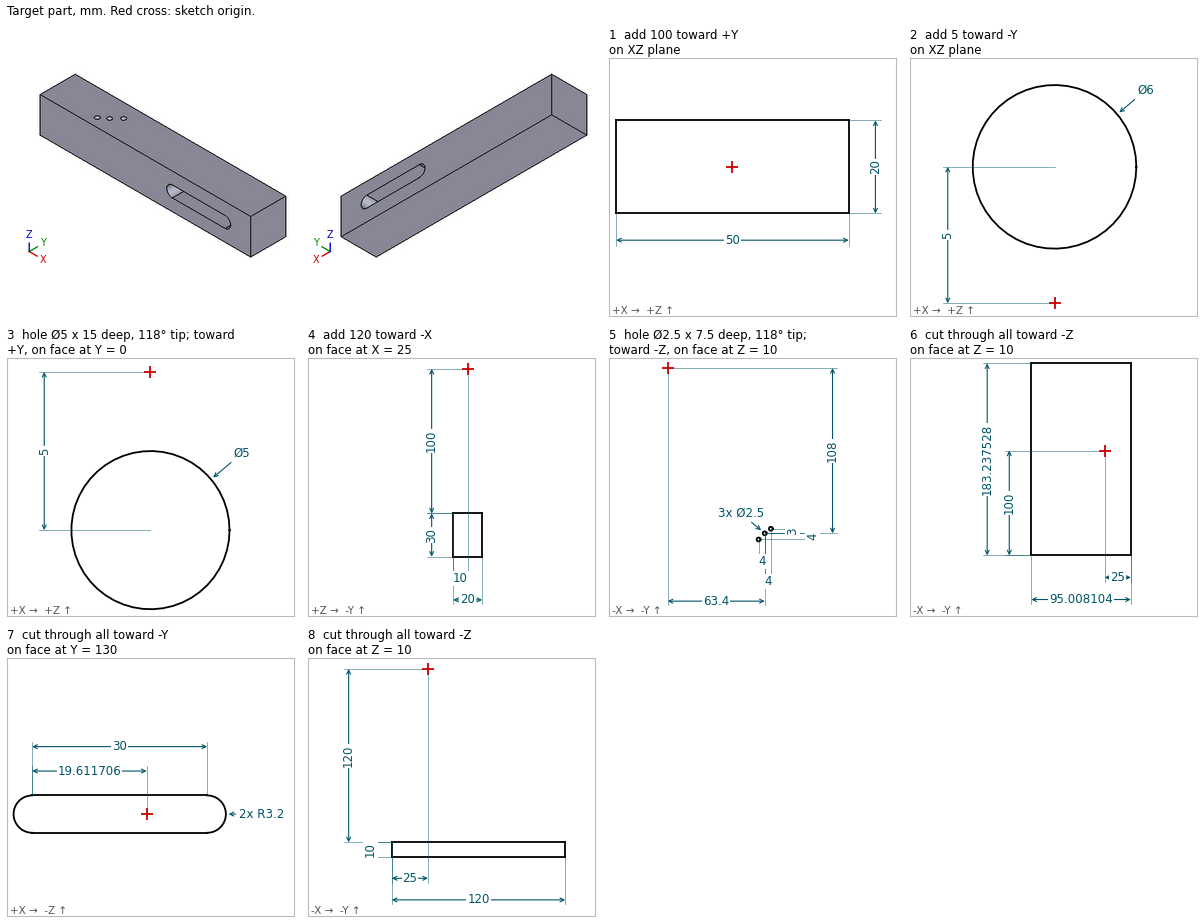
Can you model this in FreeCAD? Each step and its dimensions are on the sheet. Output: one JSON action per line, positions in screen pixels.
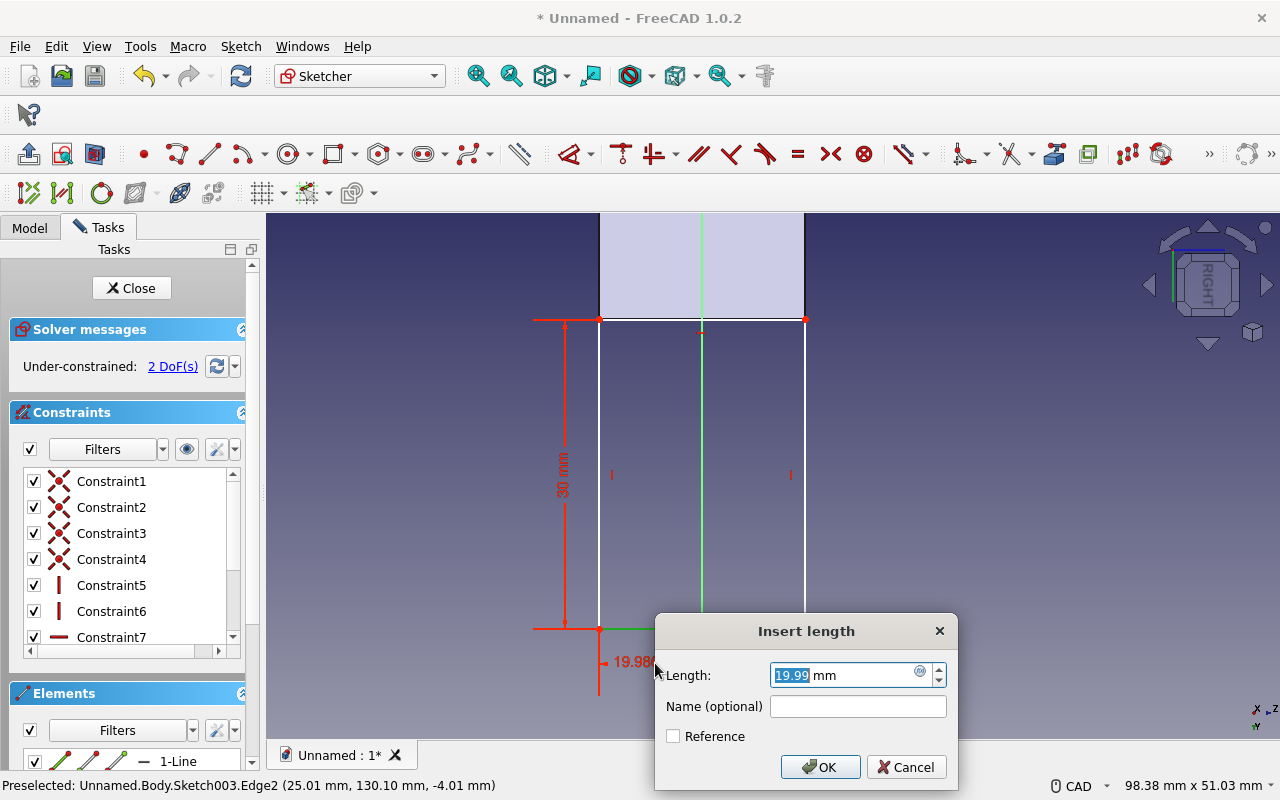
{"action": "type", "text": "20"}
{"action": "key", "text": "Return"}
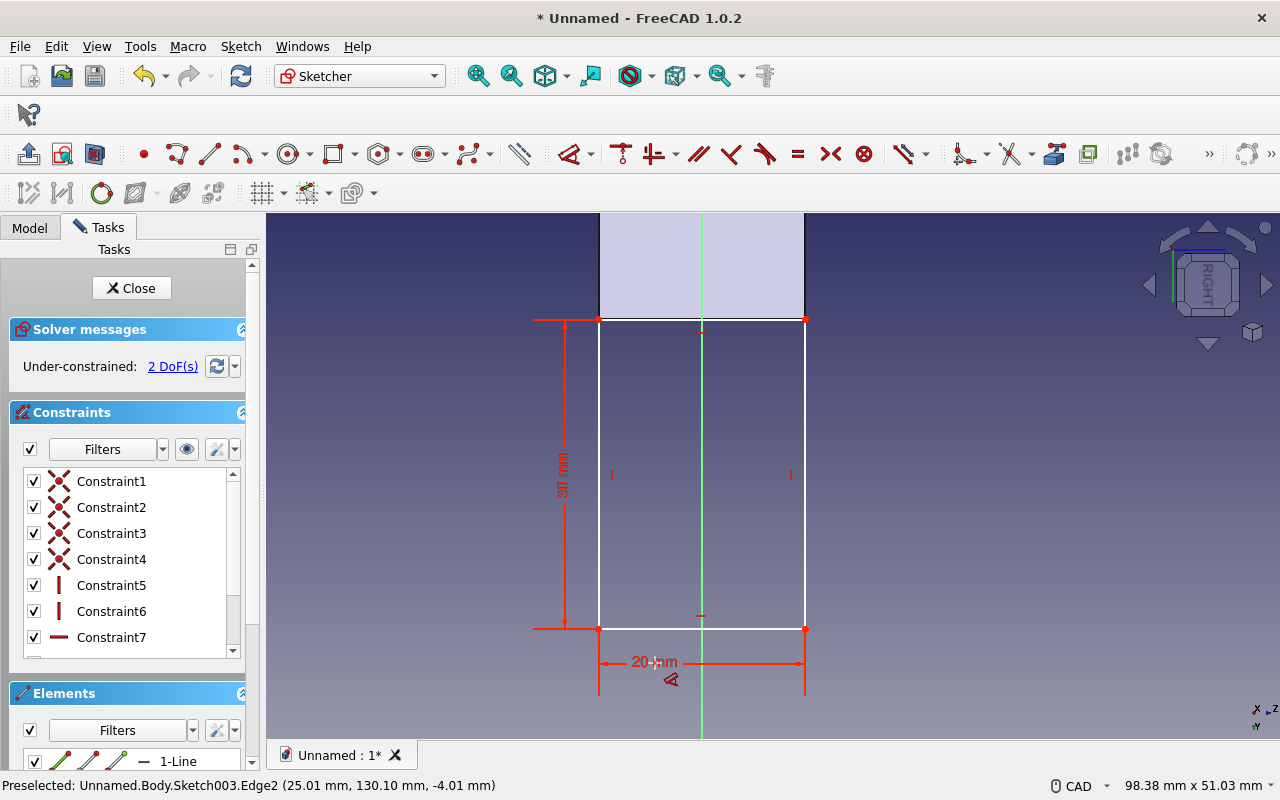
{"action": "left_click", "coordinate": [599, 320]}
{"action": "left_click", "coordinate": [651, 354]}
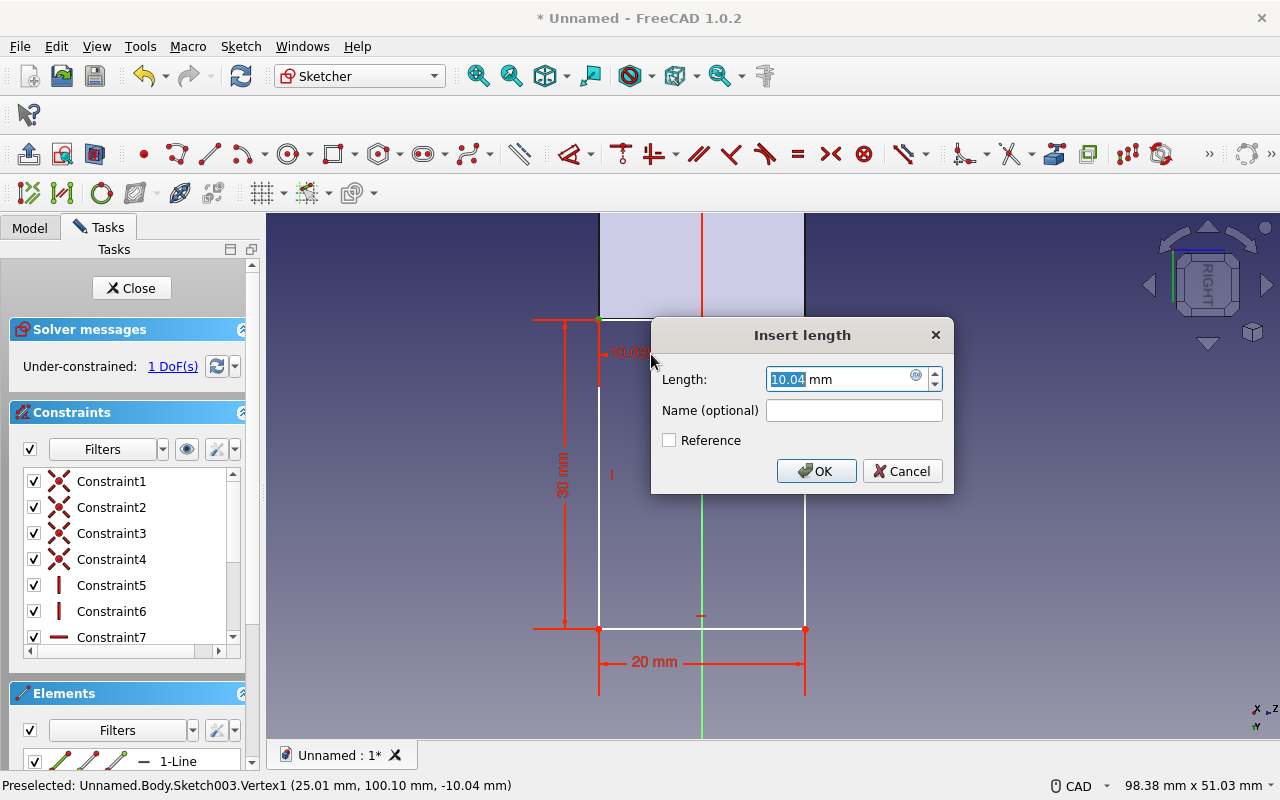
{"action": "type", "text": "10"}
{"action": "key", "text": "Return"}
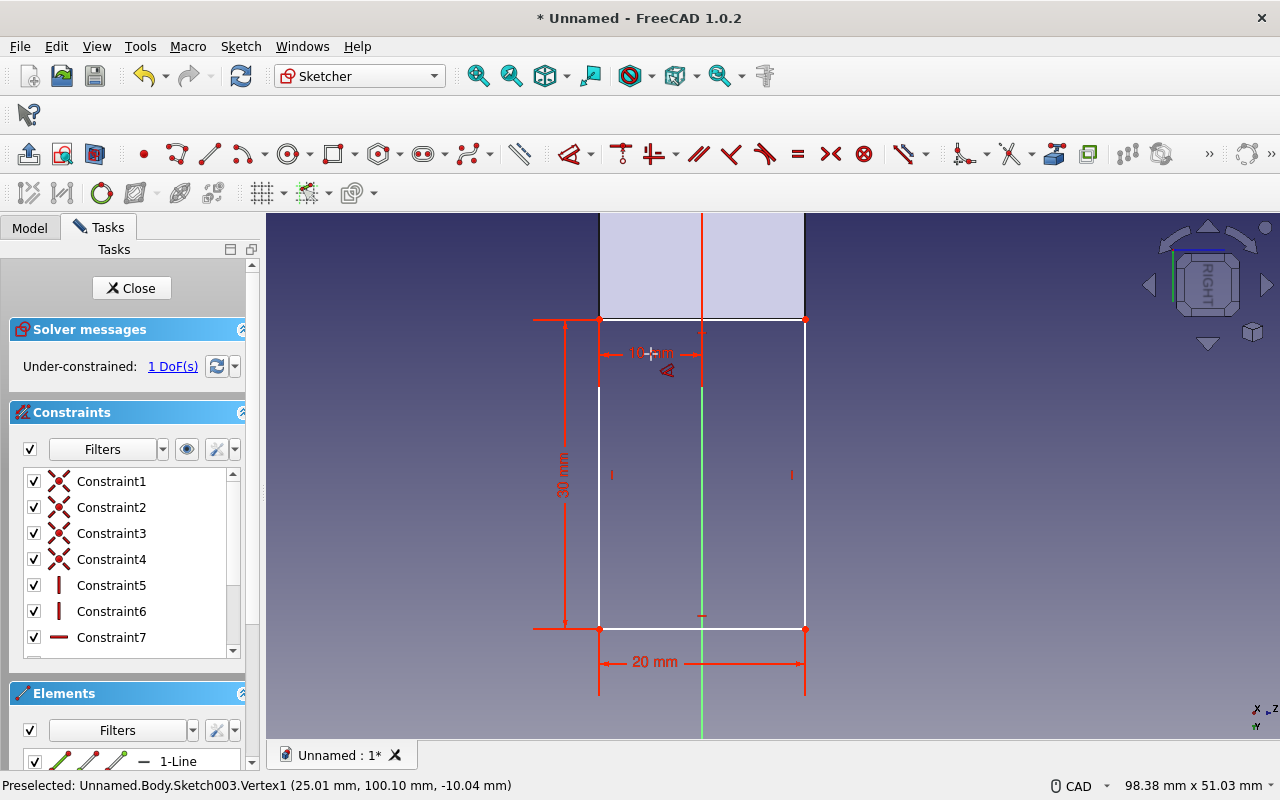
{"action": "left_click", "coordinate": [599, 320]}
{"action": "left_click", "coordinate": [565, 280]}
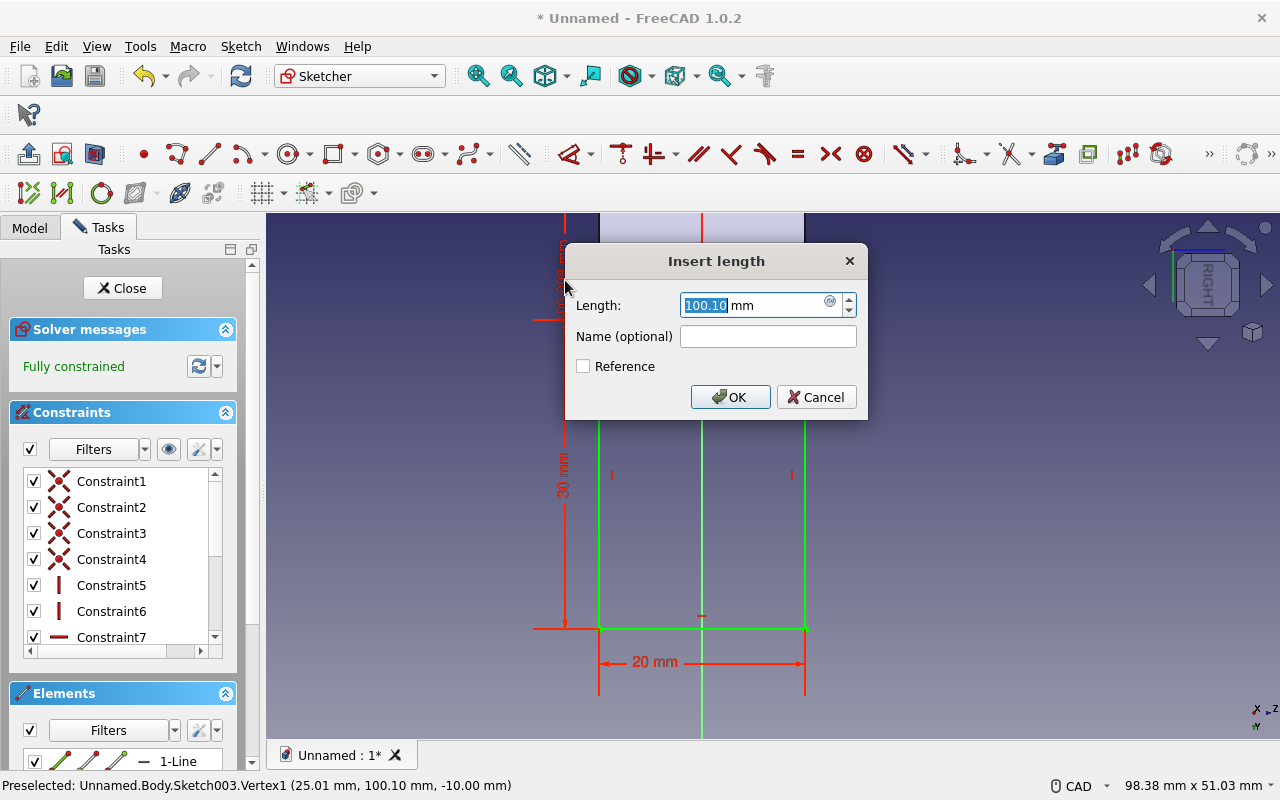
{"action": "type", "text": "100"}
{"action": "key", "text": "Return"}
{"action": "key", "text": "Escape"}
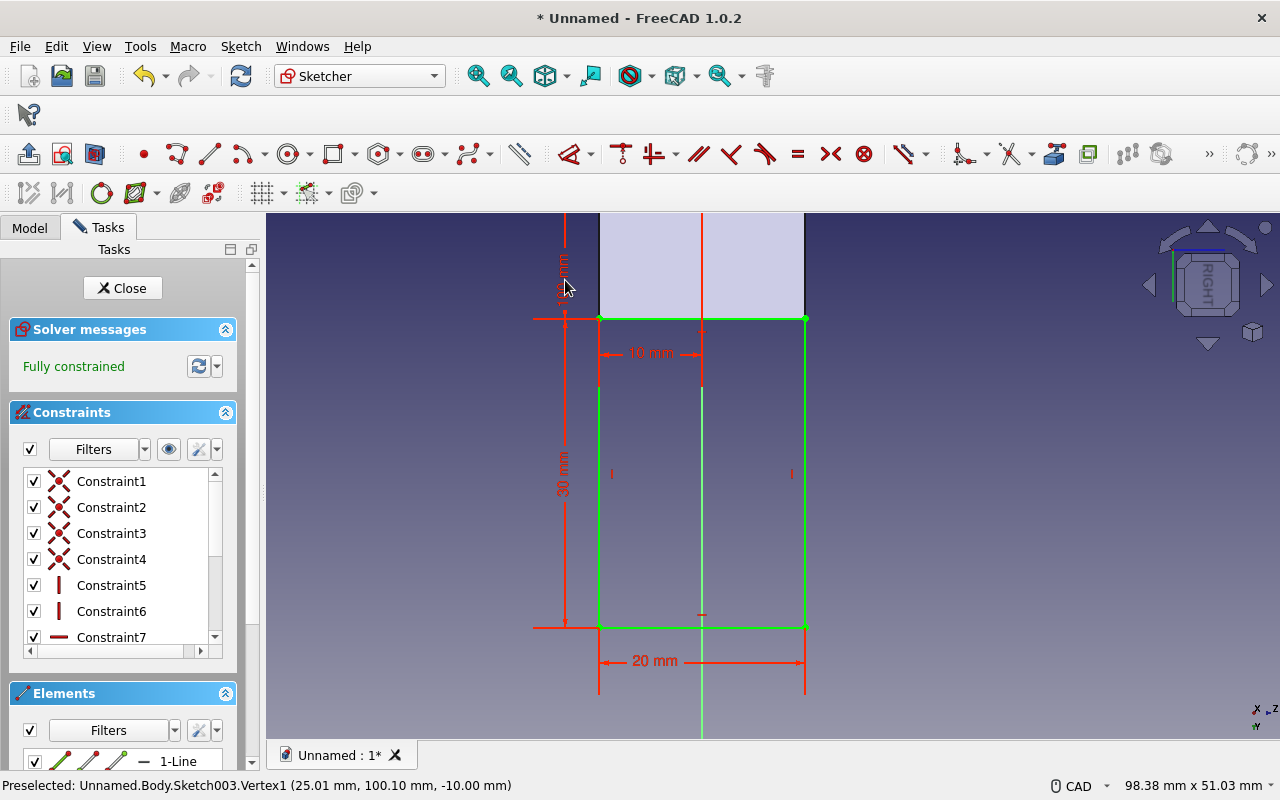
{"action": "left_click", "coordinate": [123, 288]}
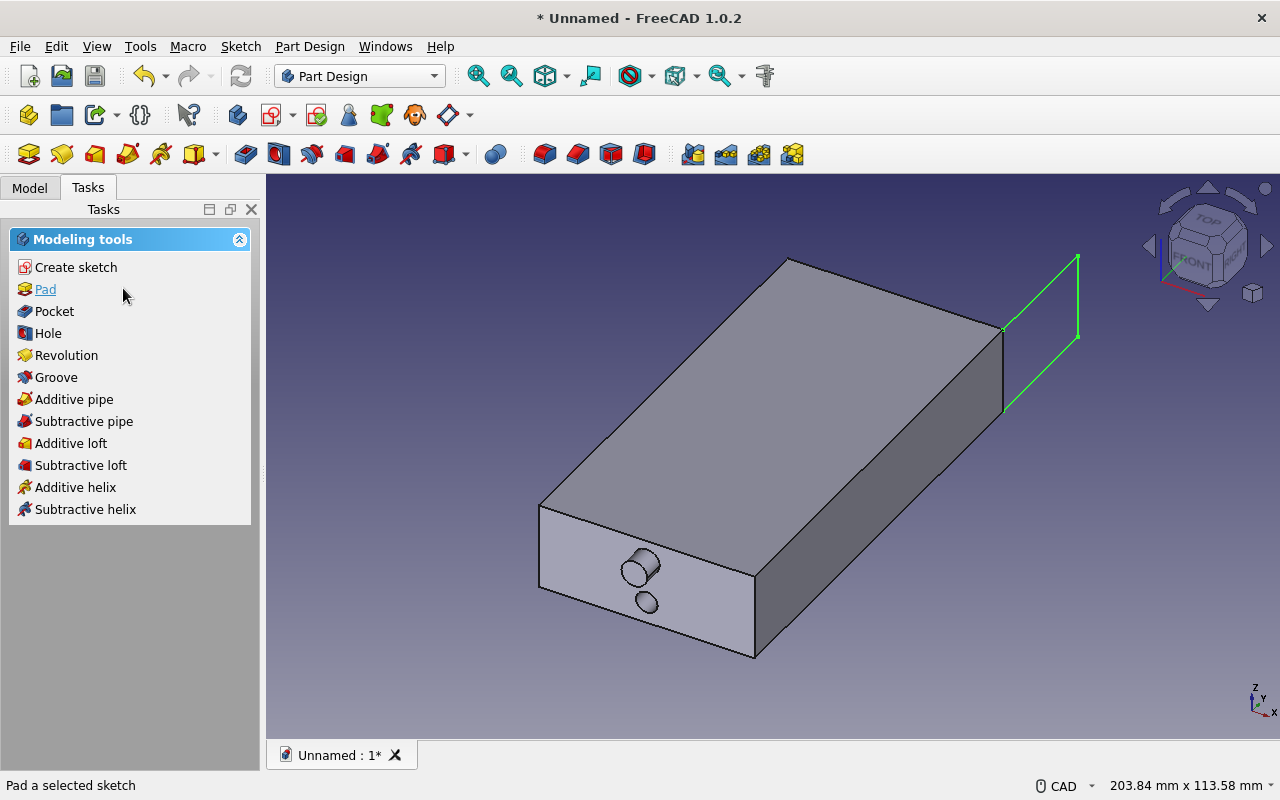
{"action": "left_click", "coordinate": [29, 154]}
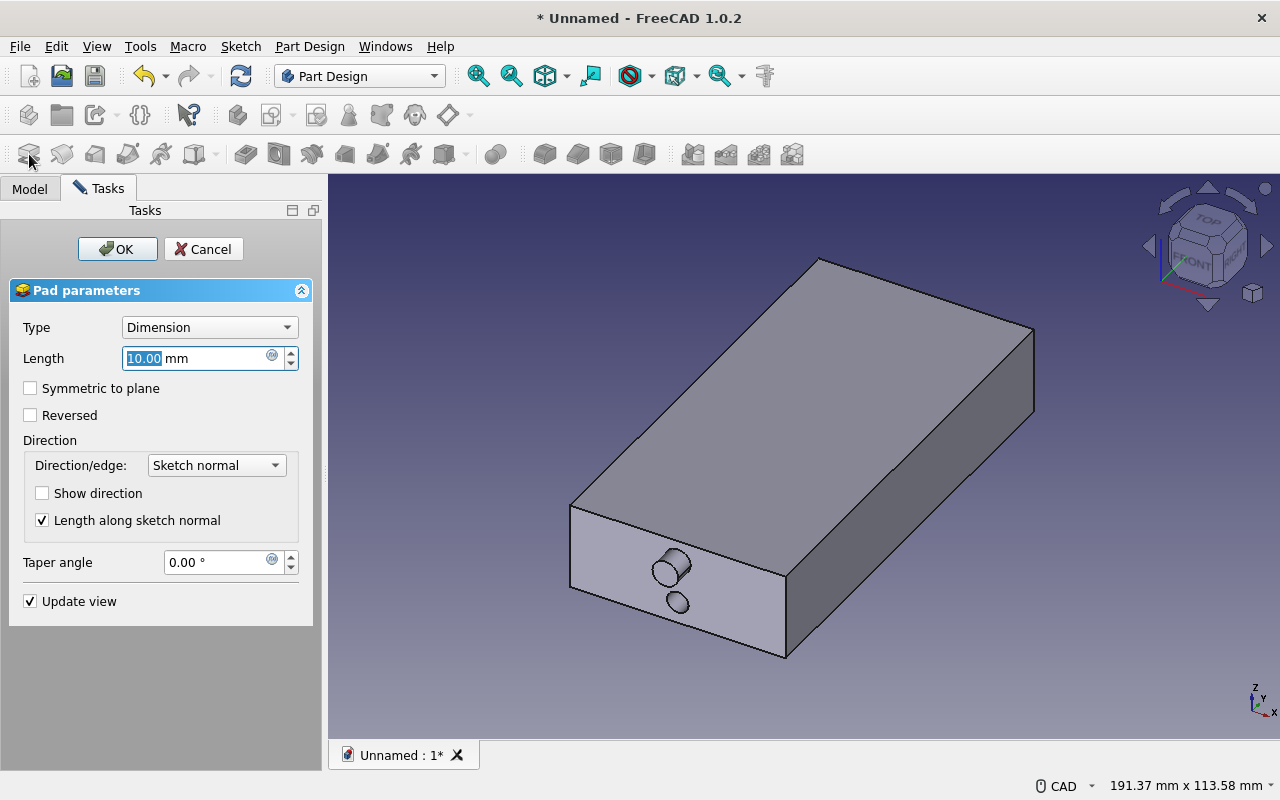
{"action": "type", "text": "120"}
{"action": "key", "text": "Tab"}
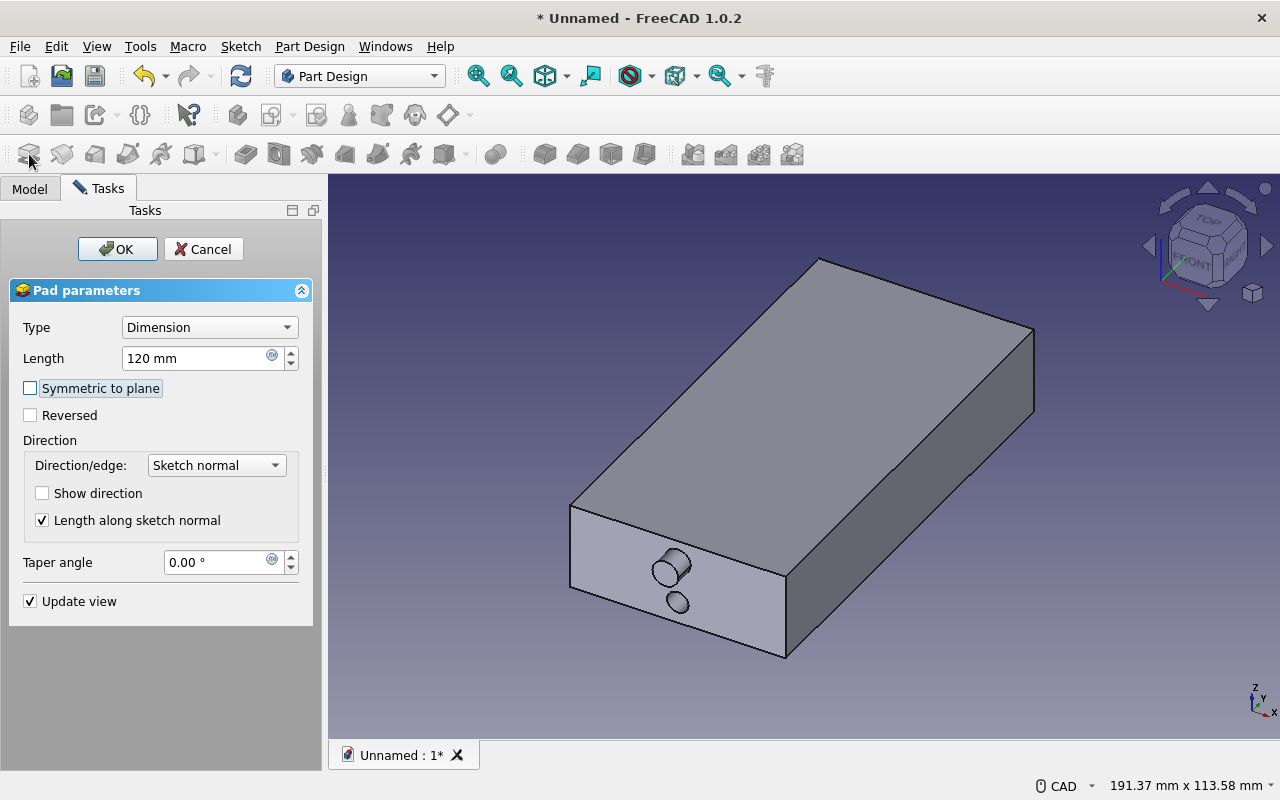
{"action": "left_click", "coordinate": [31, 415]}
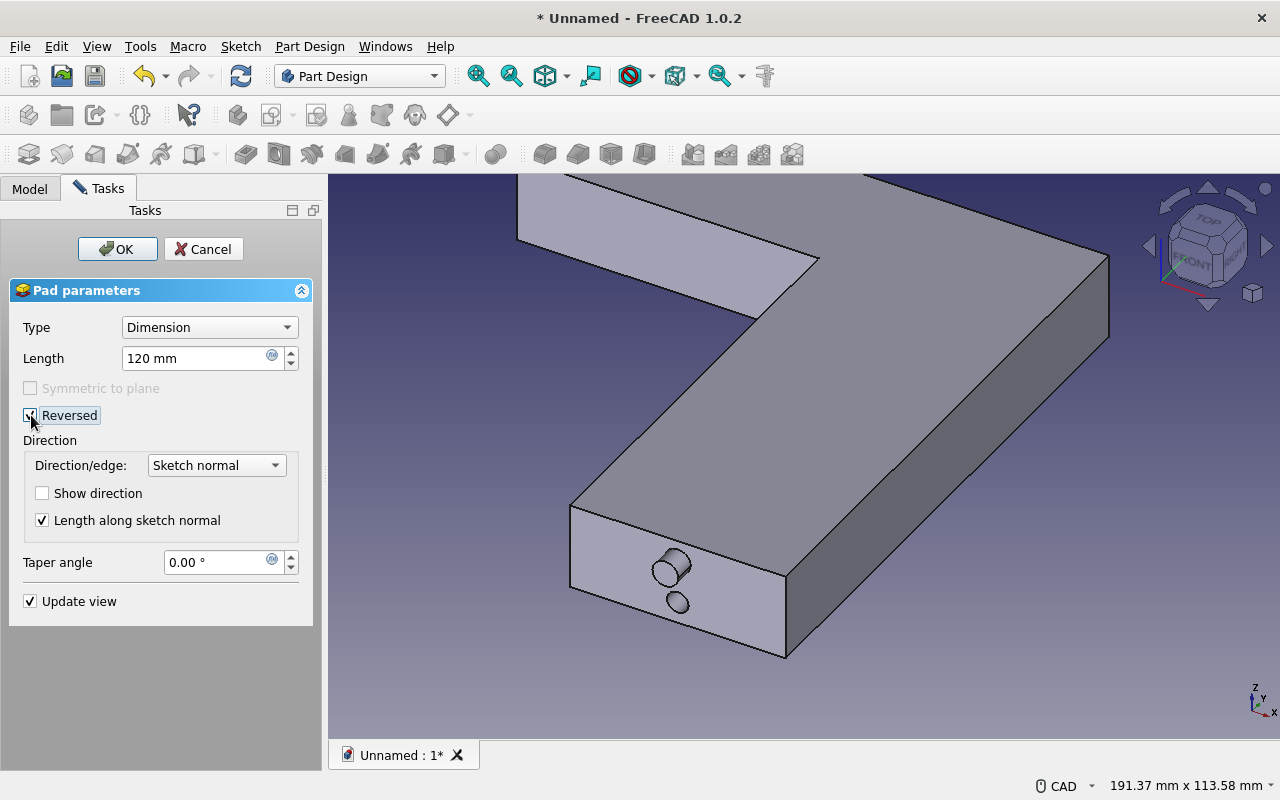
{"action": "left_click", "coordinate": [118, 249]}